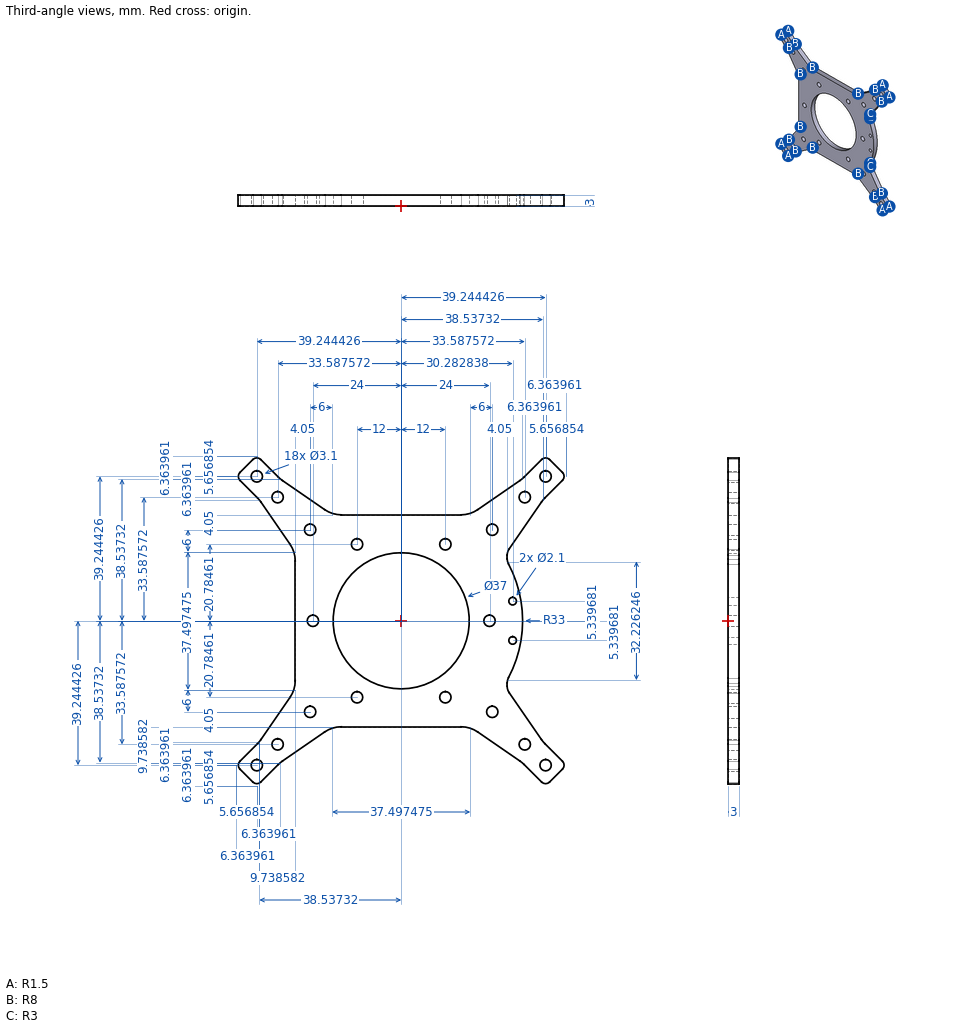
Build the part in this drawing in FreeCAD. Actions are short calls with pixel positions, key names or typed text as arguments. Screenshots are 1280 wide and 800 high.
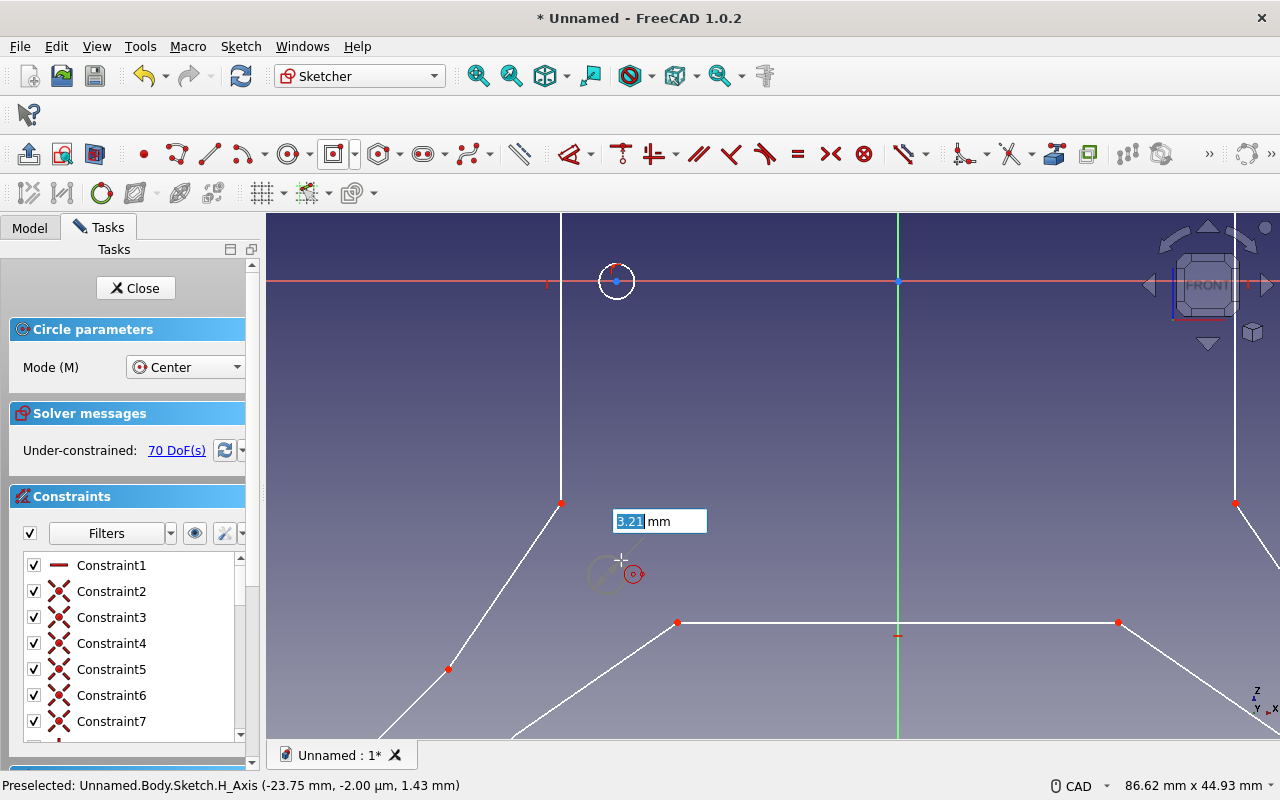
click(621, 558)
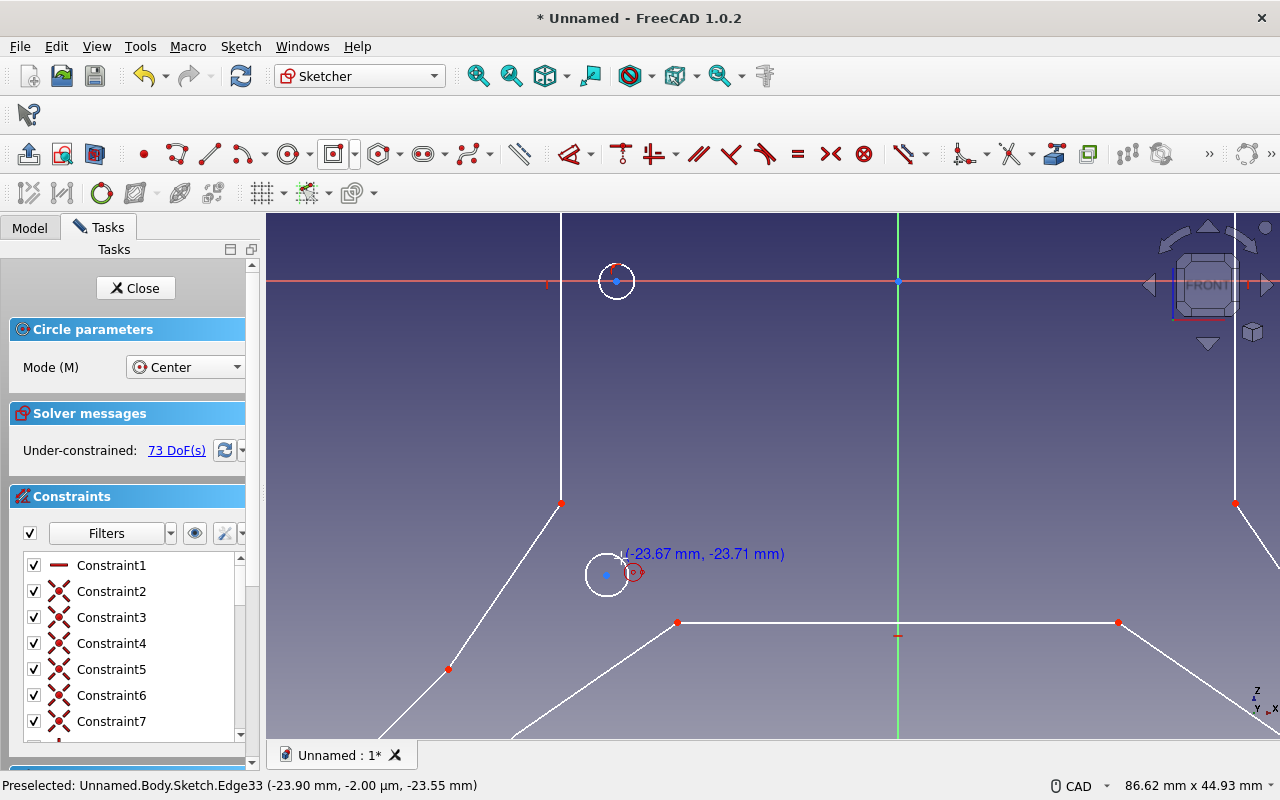
scroll(505, 675, up, 2)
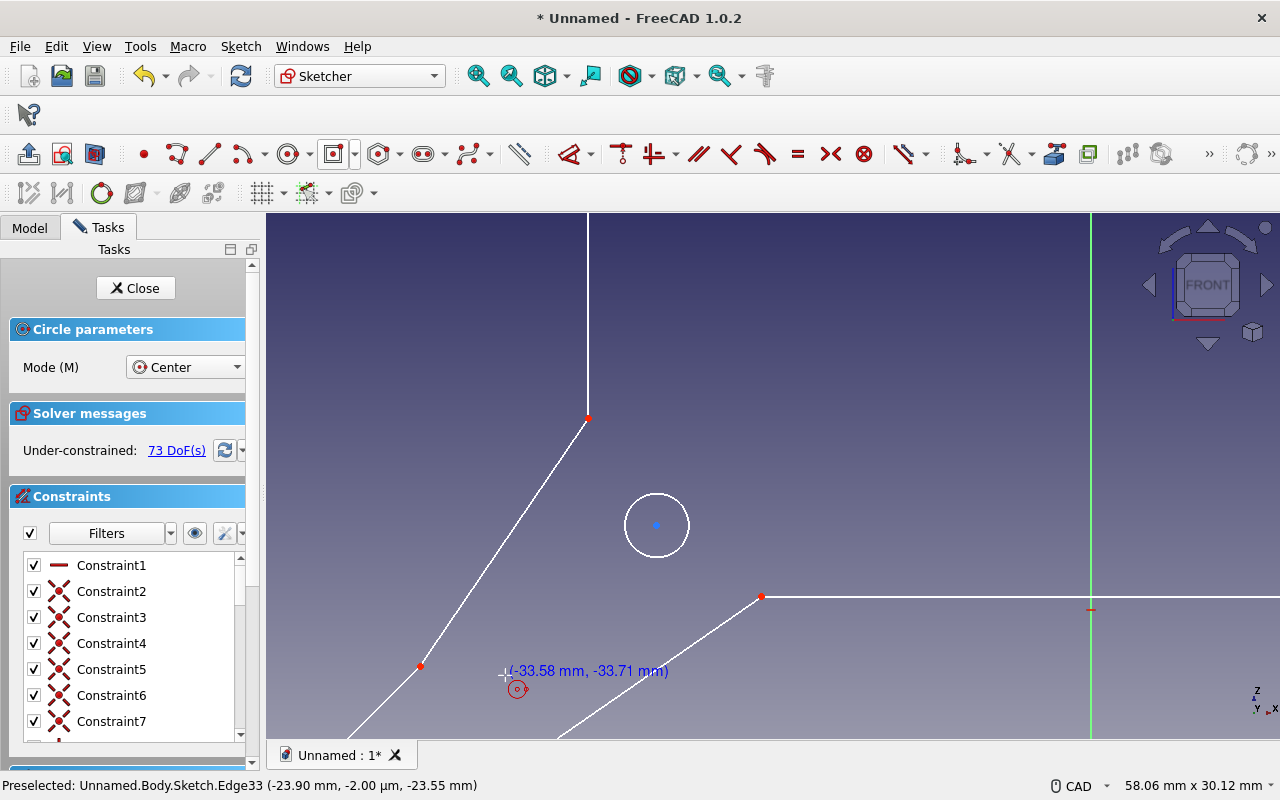
scroll(607, 574, down, 8)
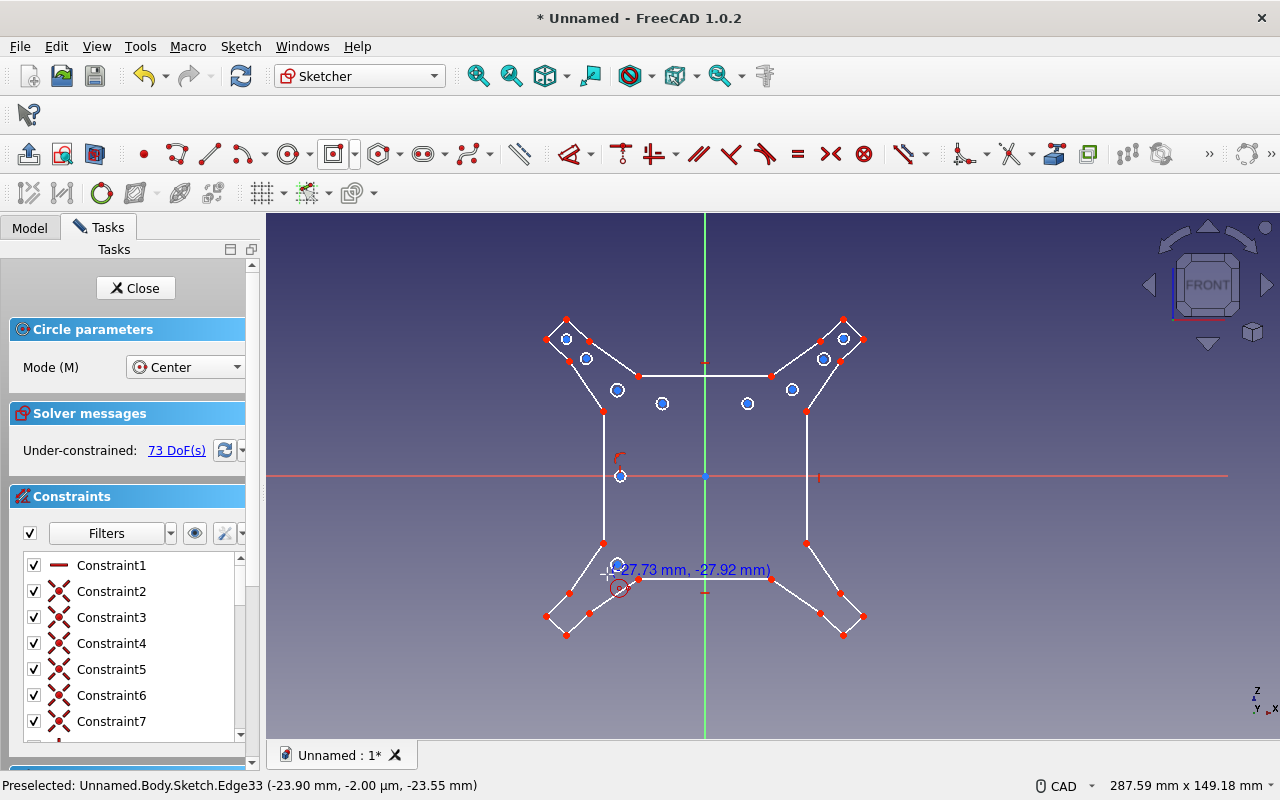
click(587, 595)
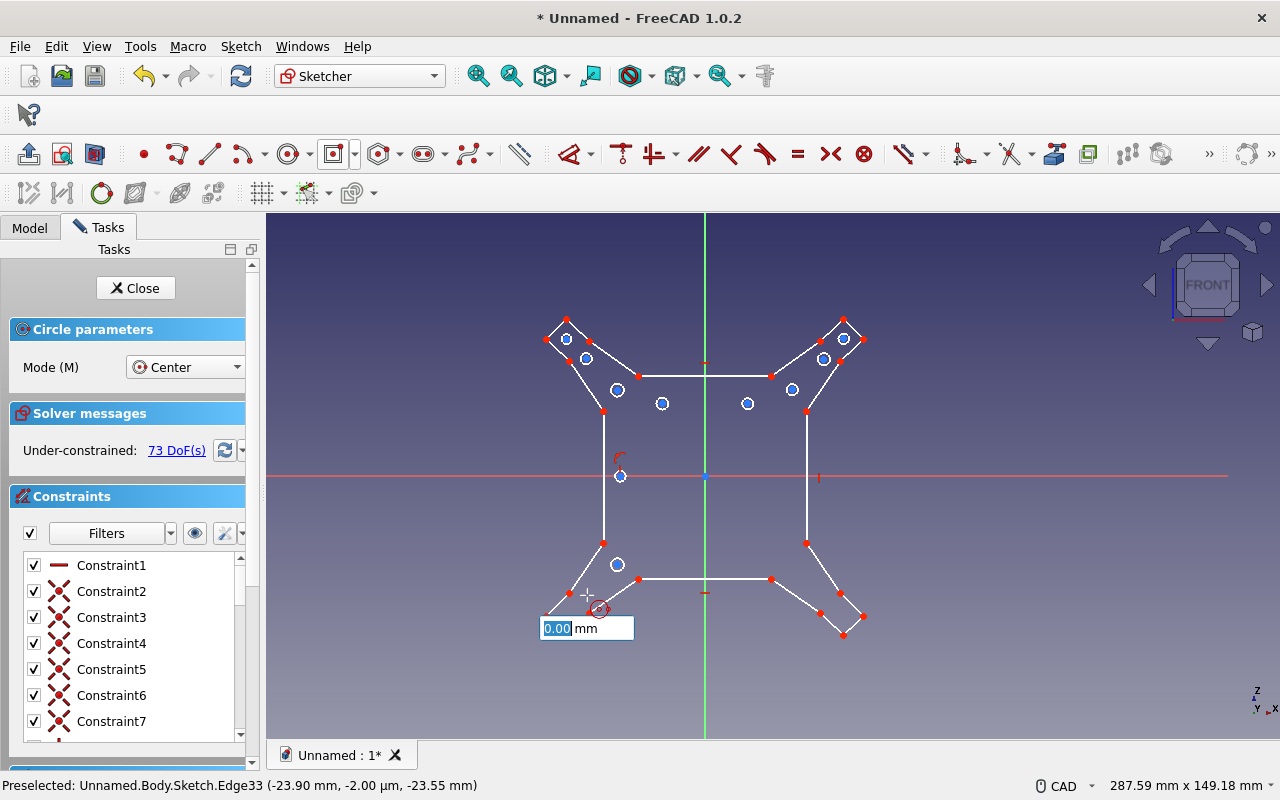
scroll(590, 591, up, 6)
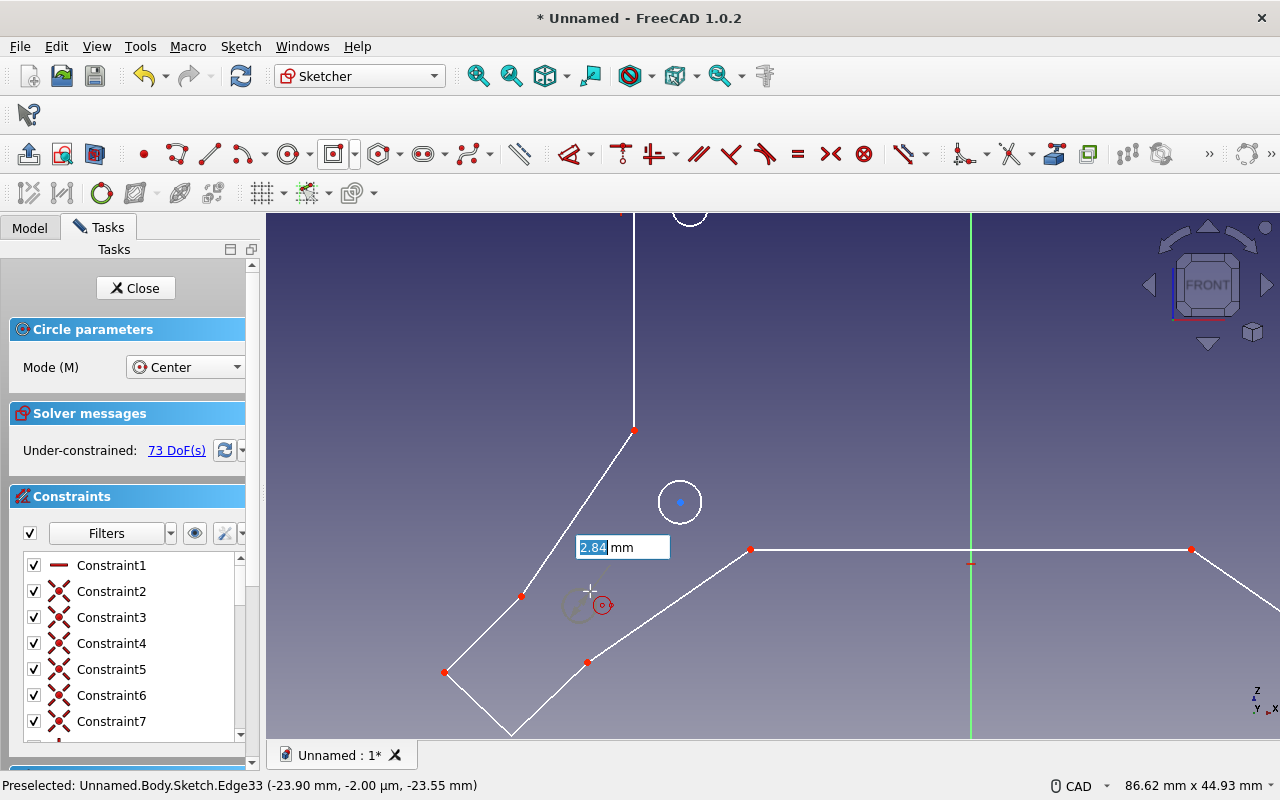
click(591, 589)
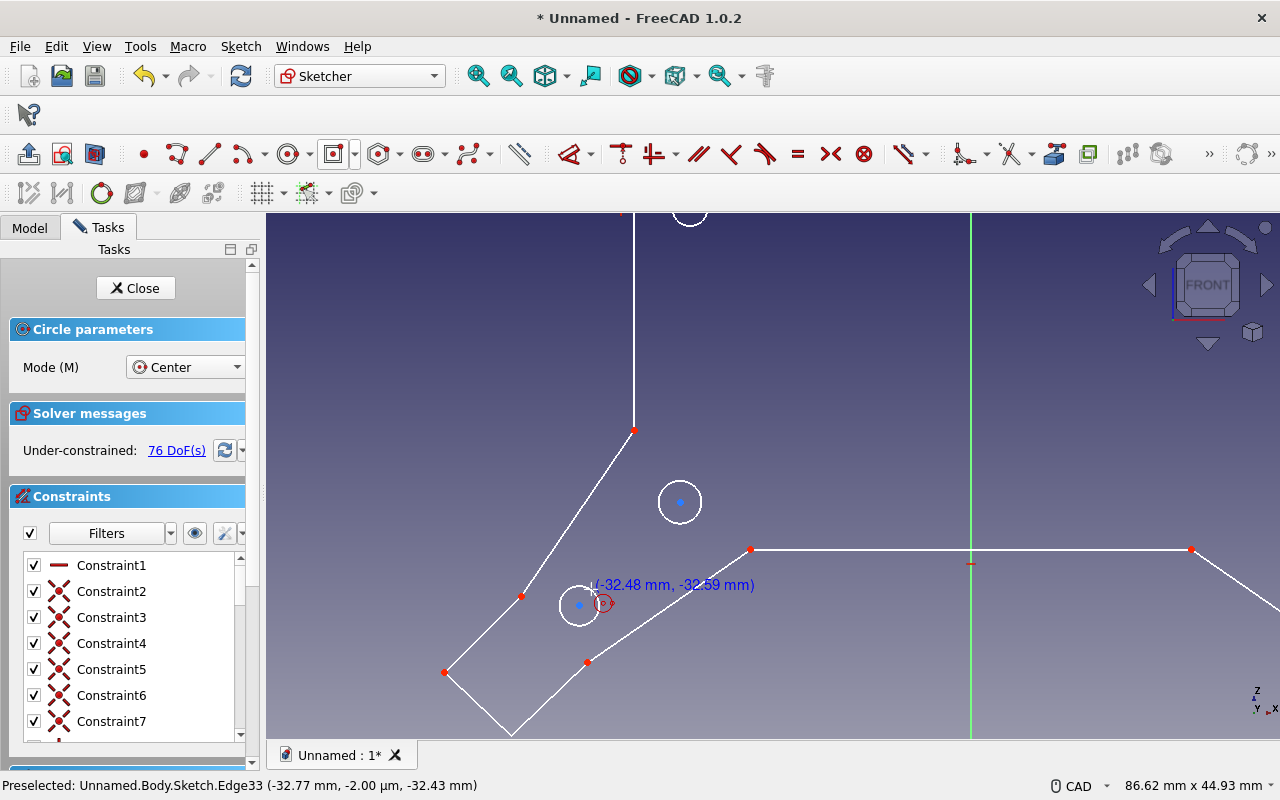
scroll(512, 668, up, 2)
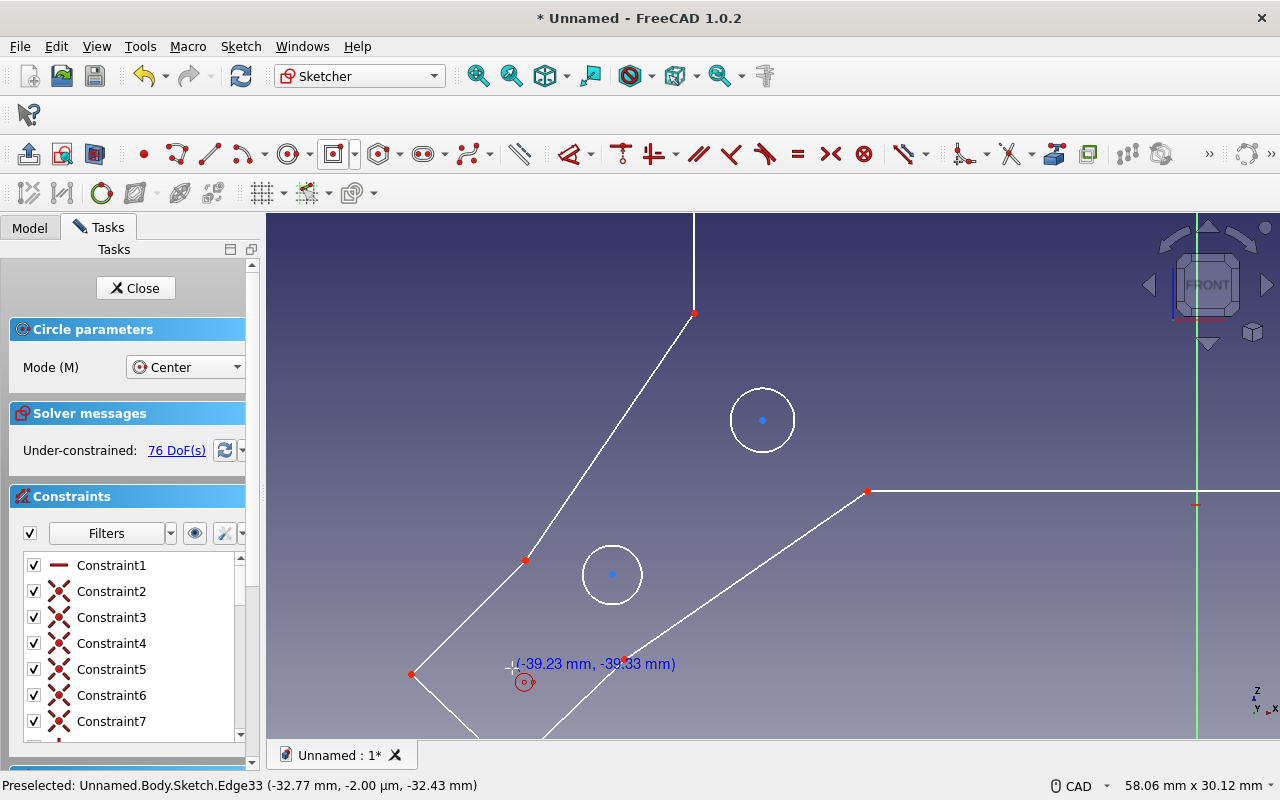
scroll(580, 601, down, 8)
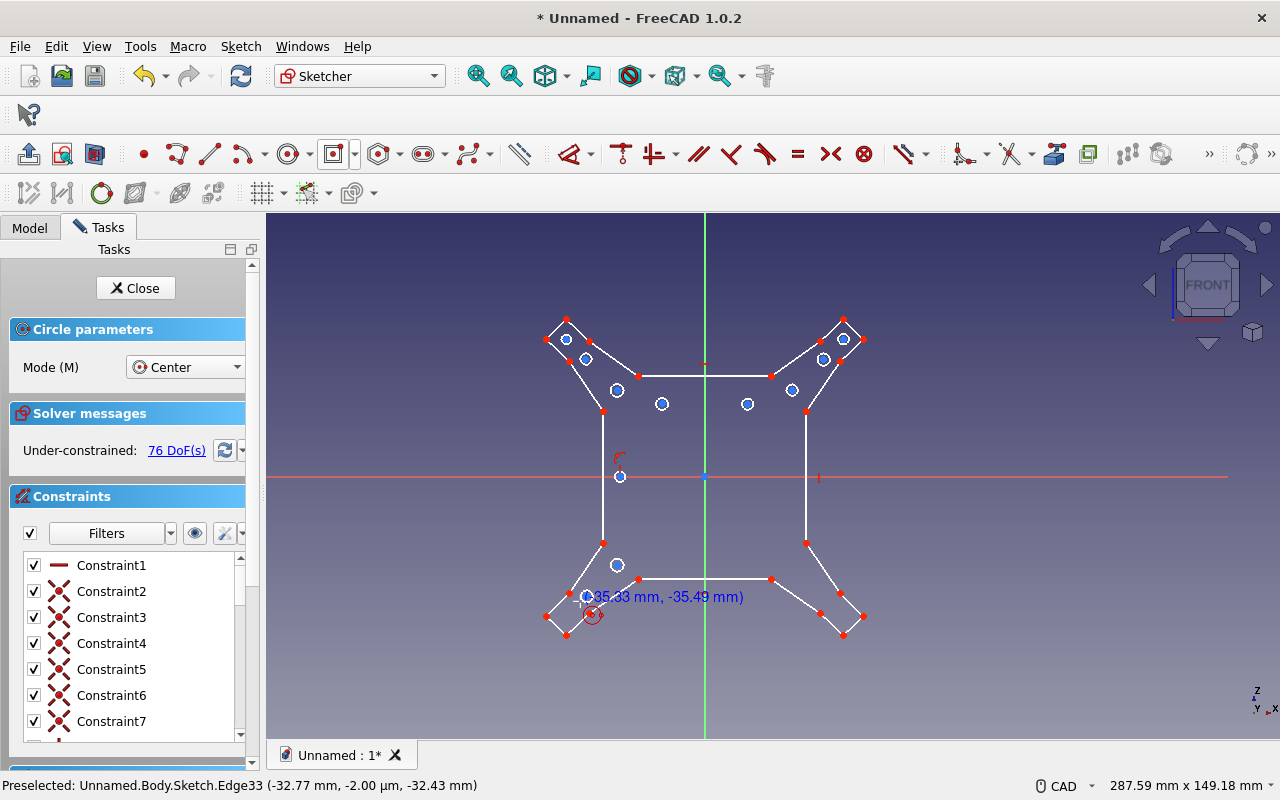
click(566, 615)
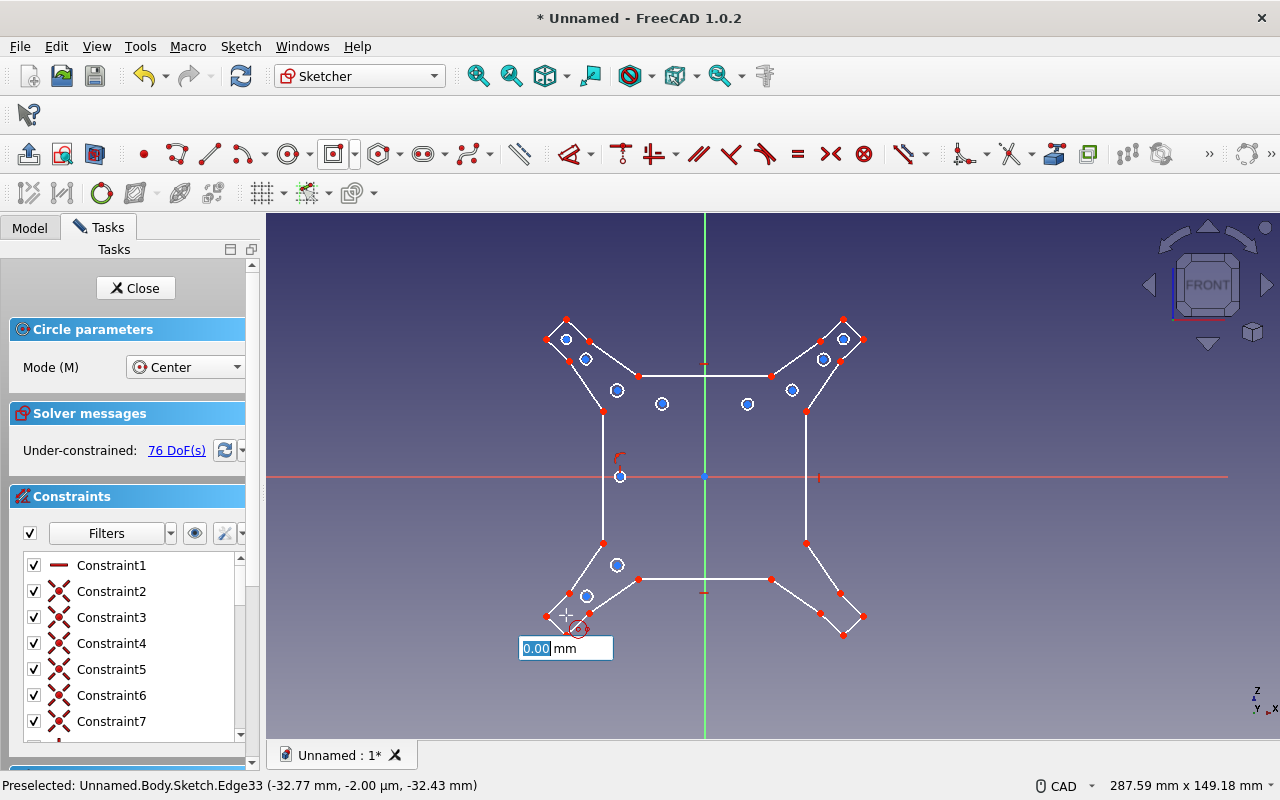
scroll(570, 611, up, 6)